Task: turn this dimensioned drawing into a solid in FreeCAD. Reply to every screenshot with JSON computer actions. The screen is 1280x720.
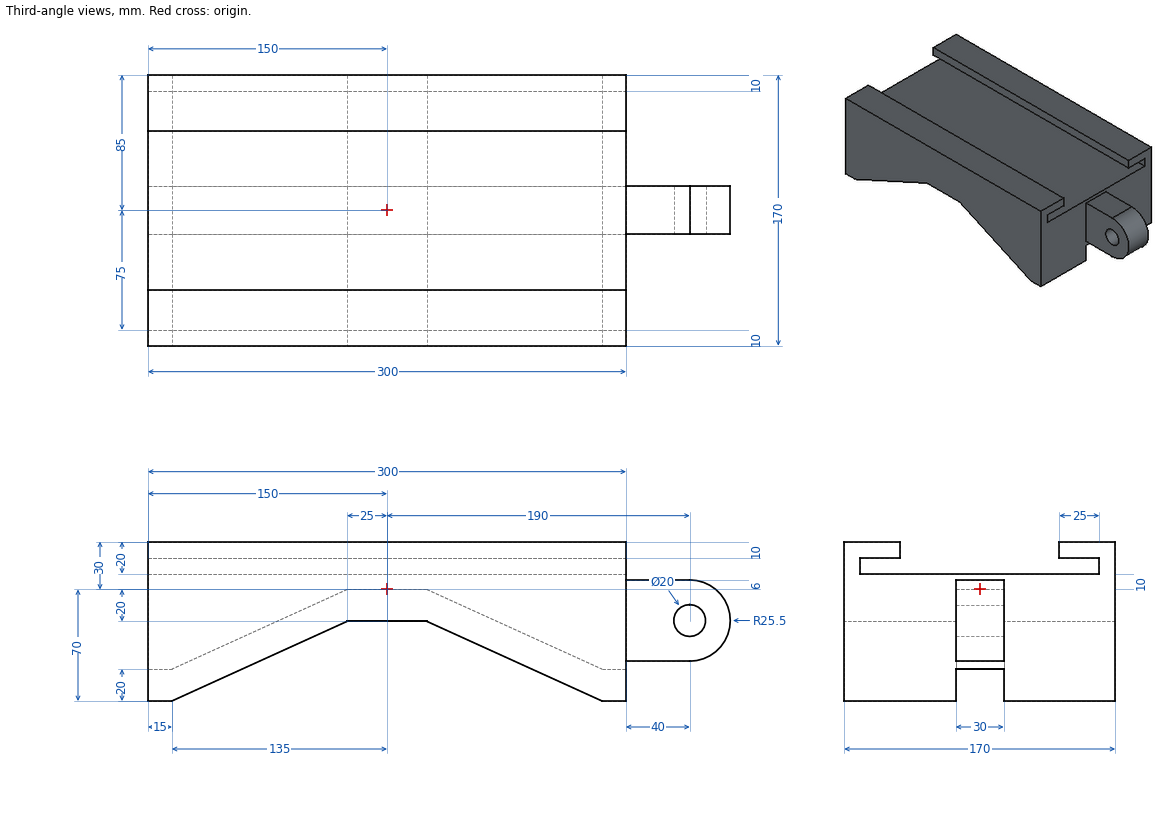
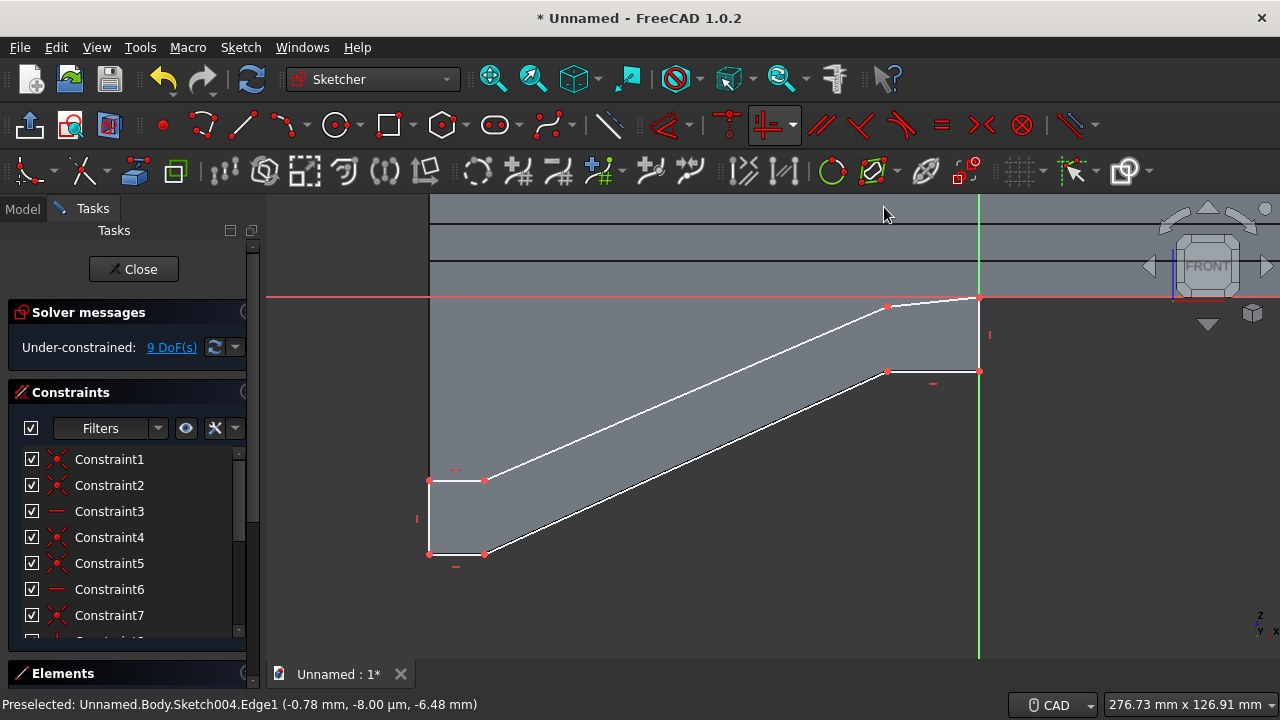
{"action": "left_click", "coordinate": [951, 300]}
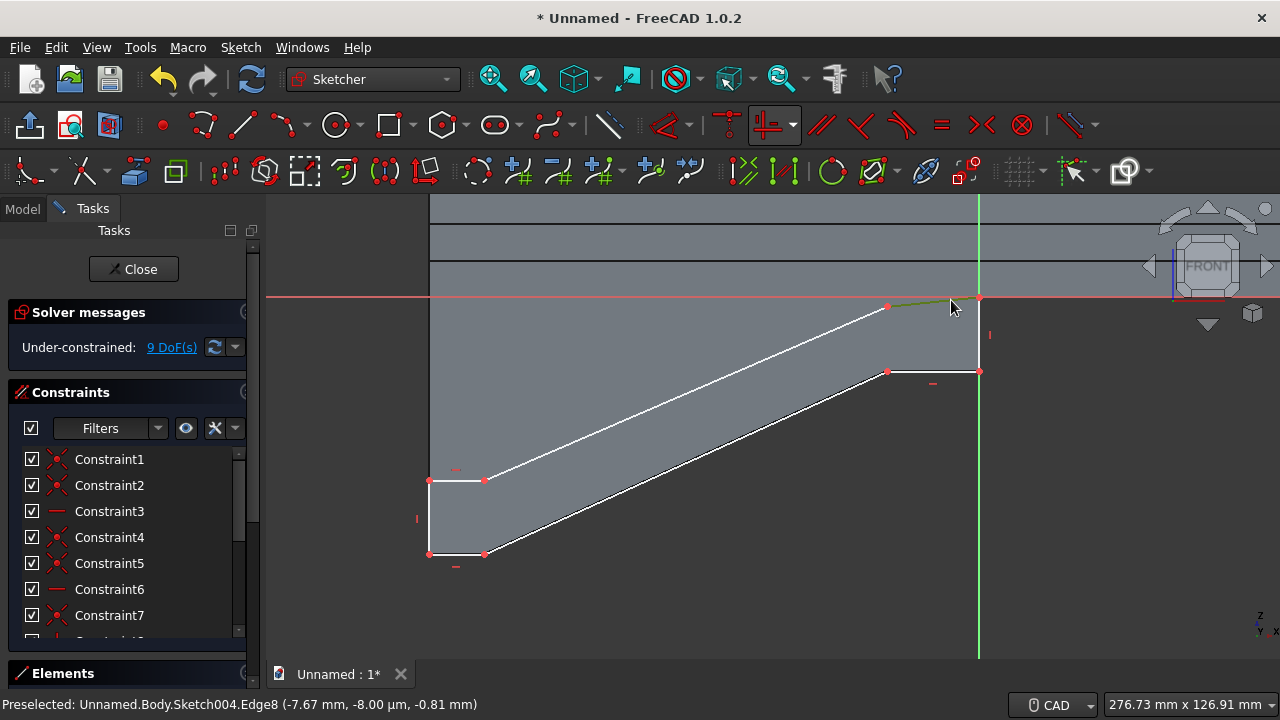
{"action": "key", "text": "h"}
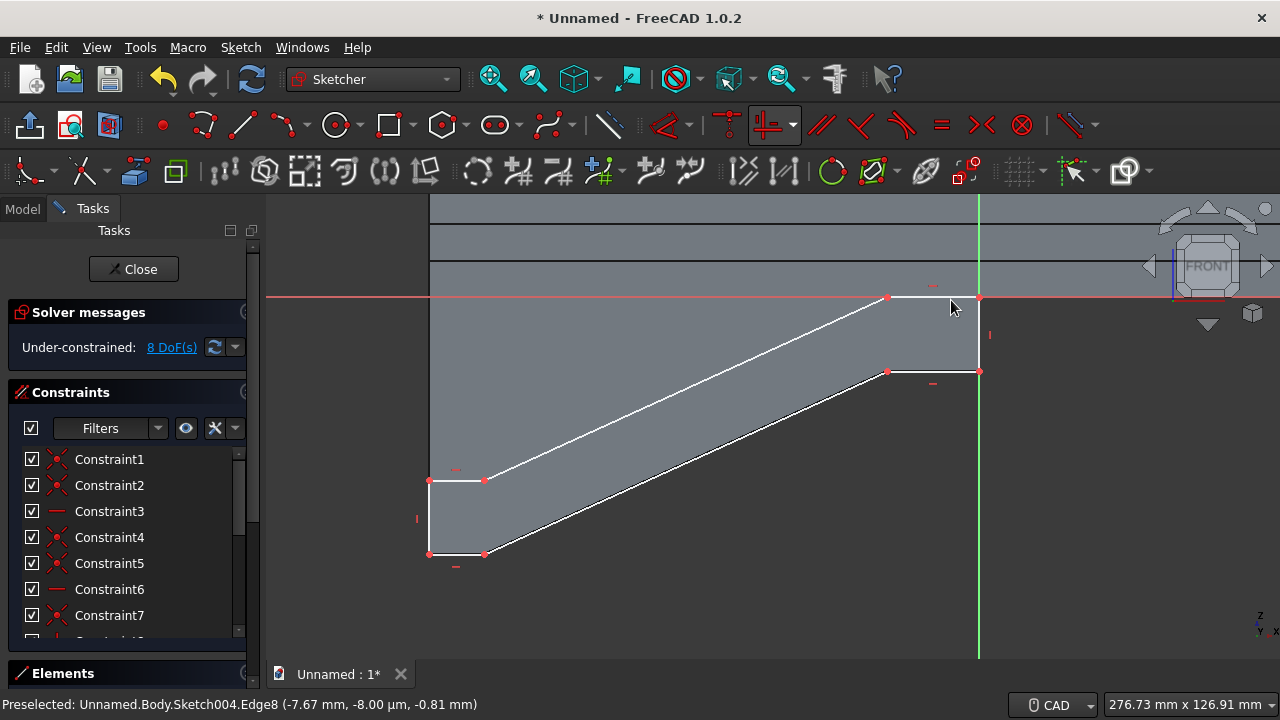
{"action": "key", "text": "d"}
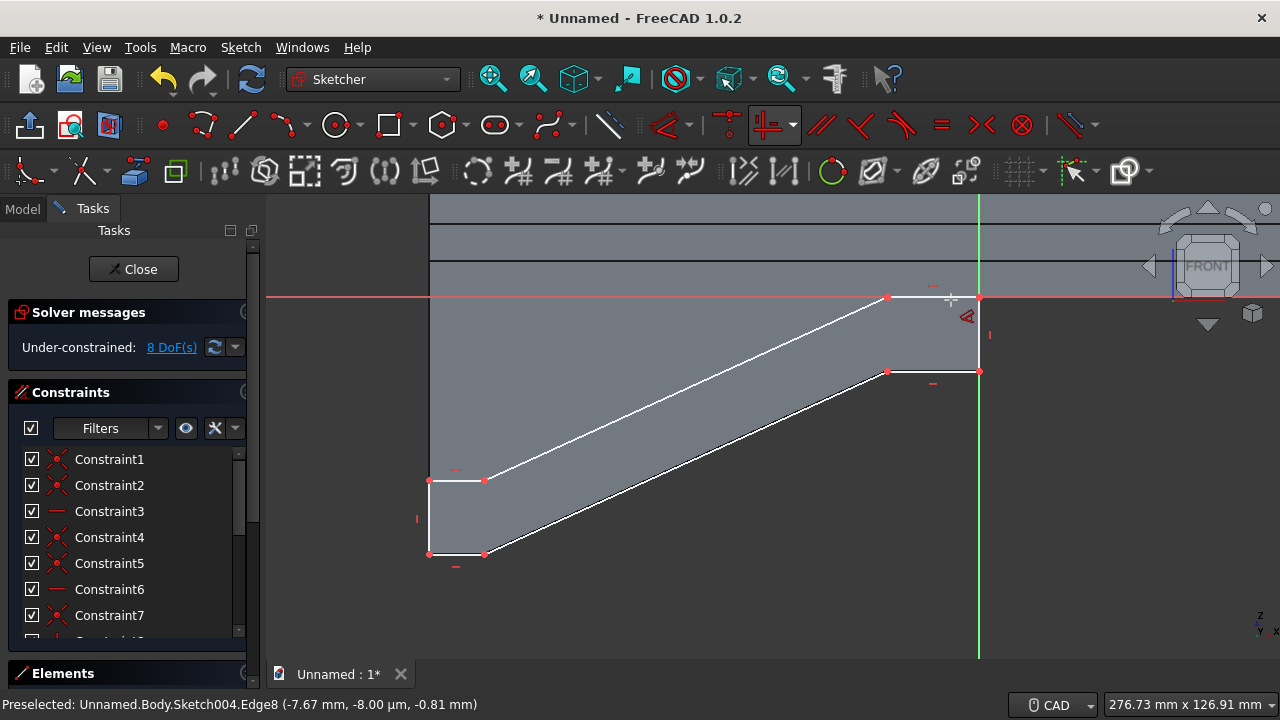
{"action": "left_click", "coordinate": [979, 320]}
{"action": "left_click", "coordinate": [1013, 335]}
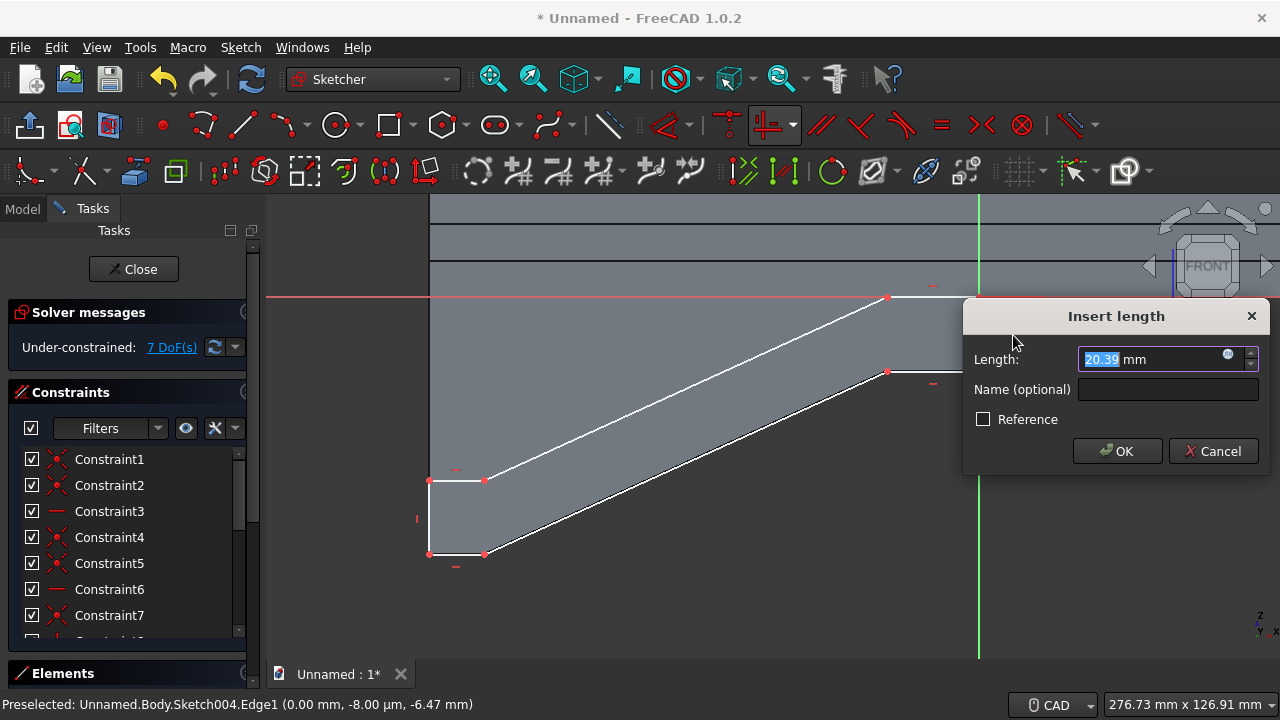
{"action": "type", "text": "20"}
{"action": "key", "text": "Return"}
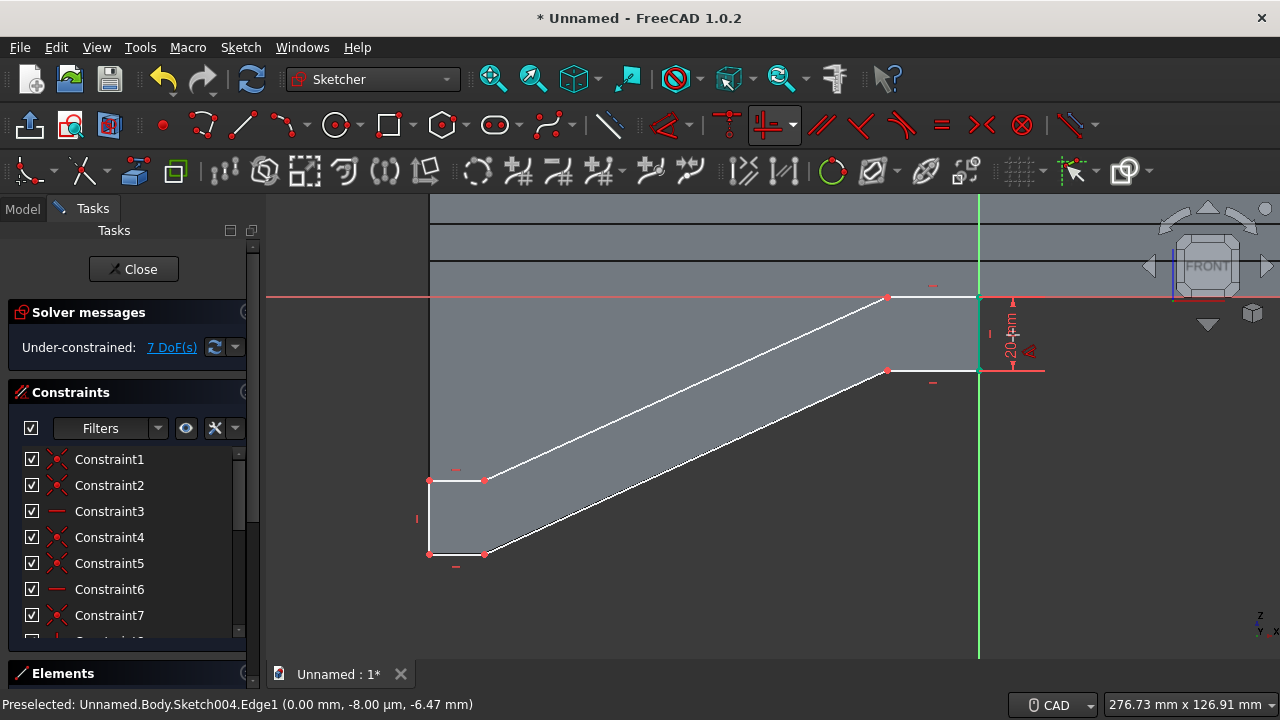
{"action": "left_click", "coordinate": [951, 371]}
{"action": "left_click", "coordinate": [933, 337]}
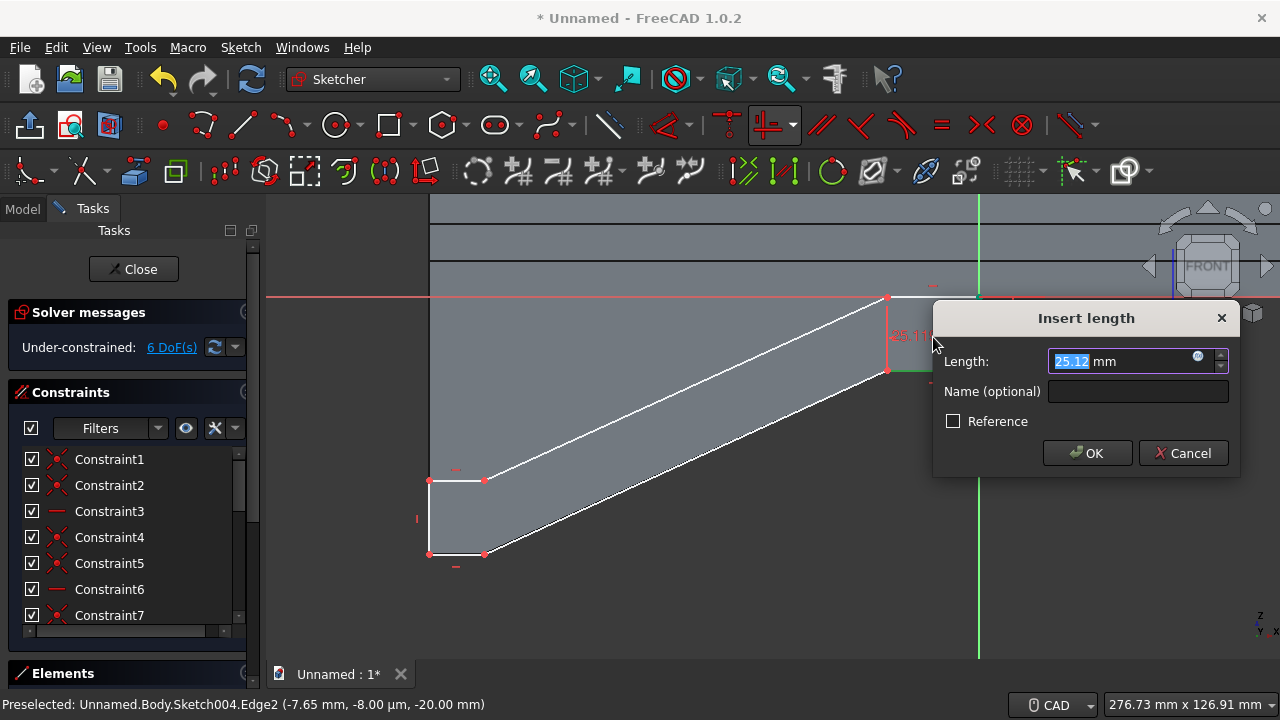
{"action": "type", "text": "25"}
{"action": "key", "text": "Return"}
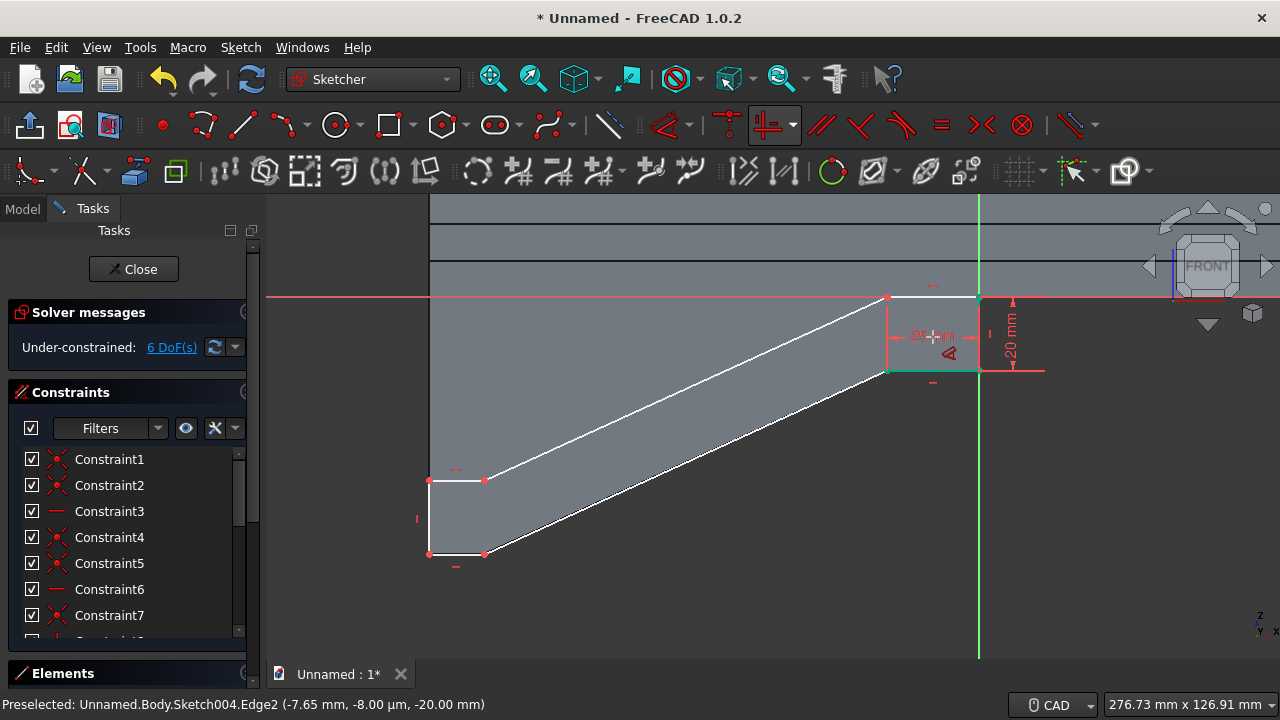
{"action": "left_click", "coordinate": [468, 555]}
{"action": "left_click", "coordinate": [457, 589]}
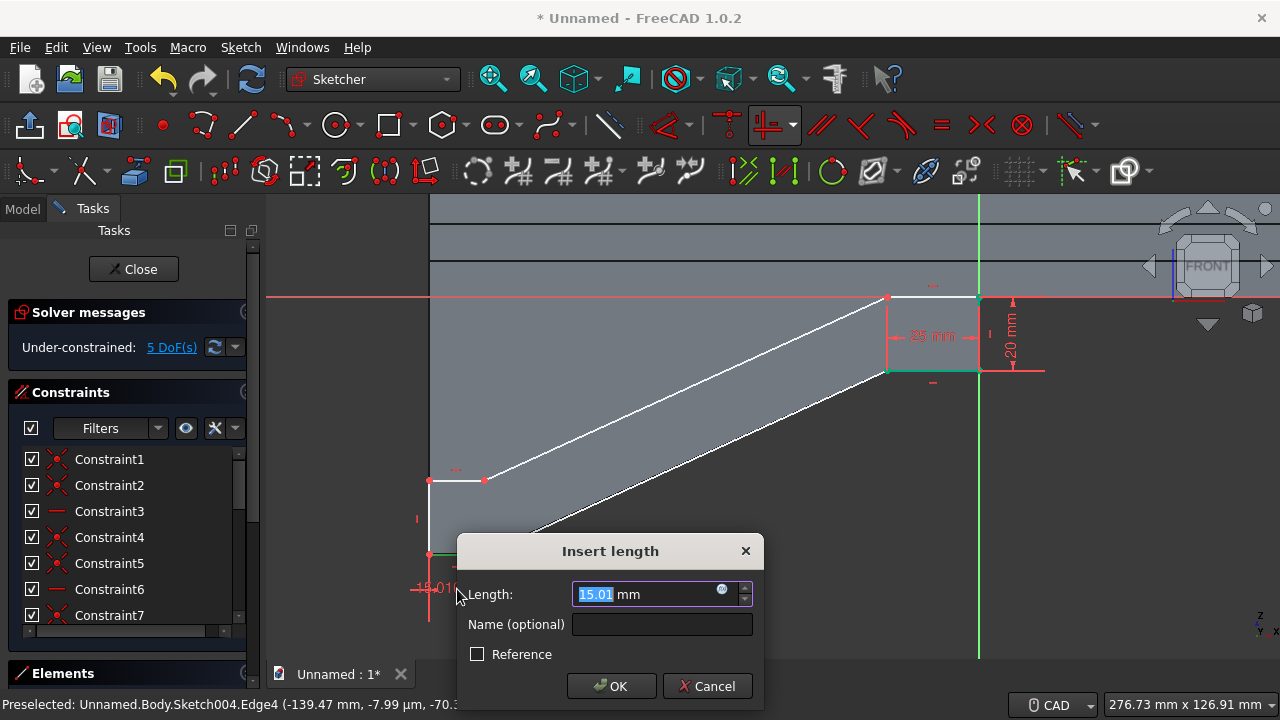
{"action": "type", "text": "15"}
{"action": "key", "text": "Return"}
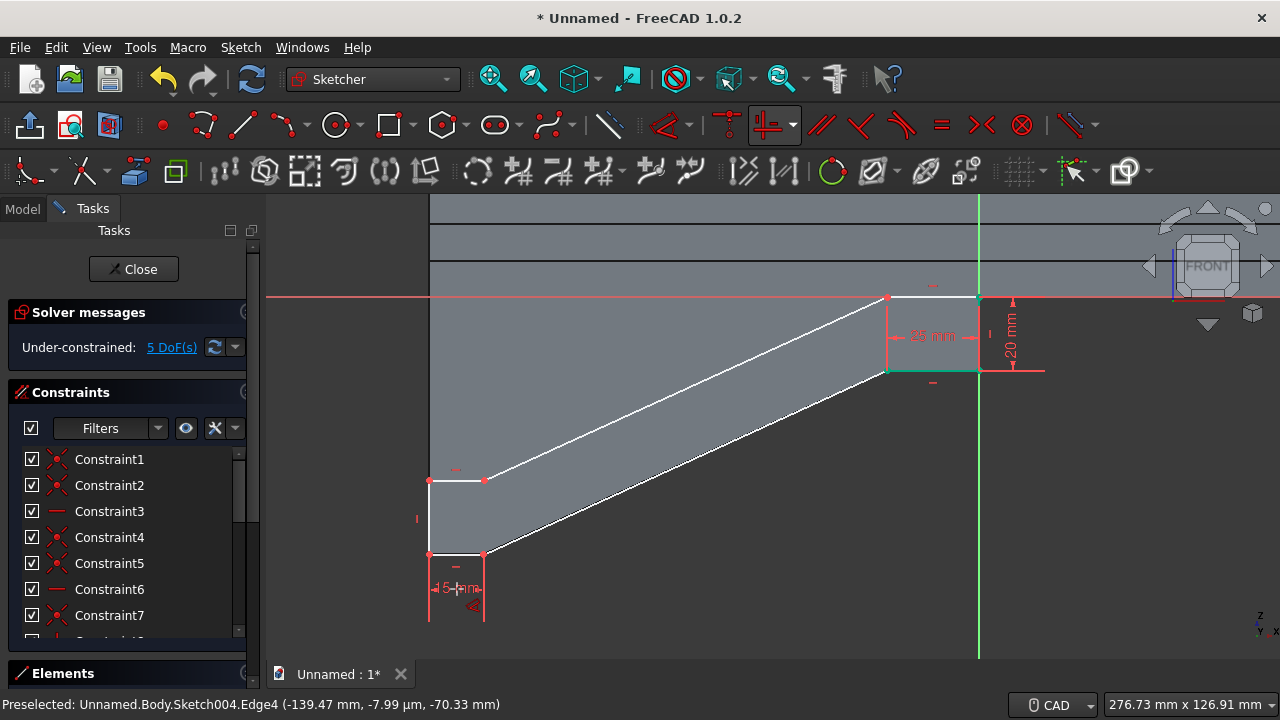
{"action": "left_click", "coordinate": [429, 533]}
{"action": "left_click", "coordinate": [395, 518]}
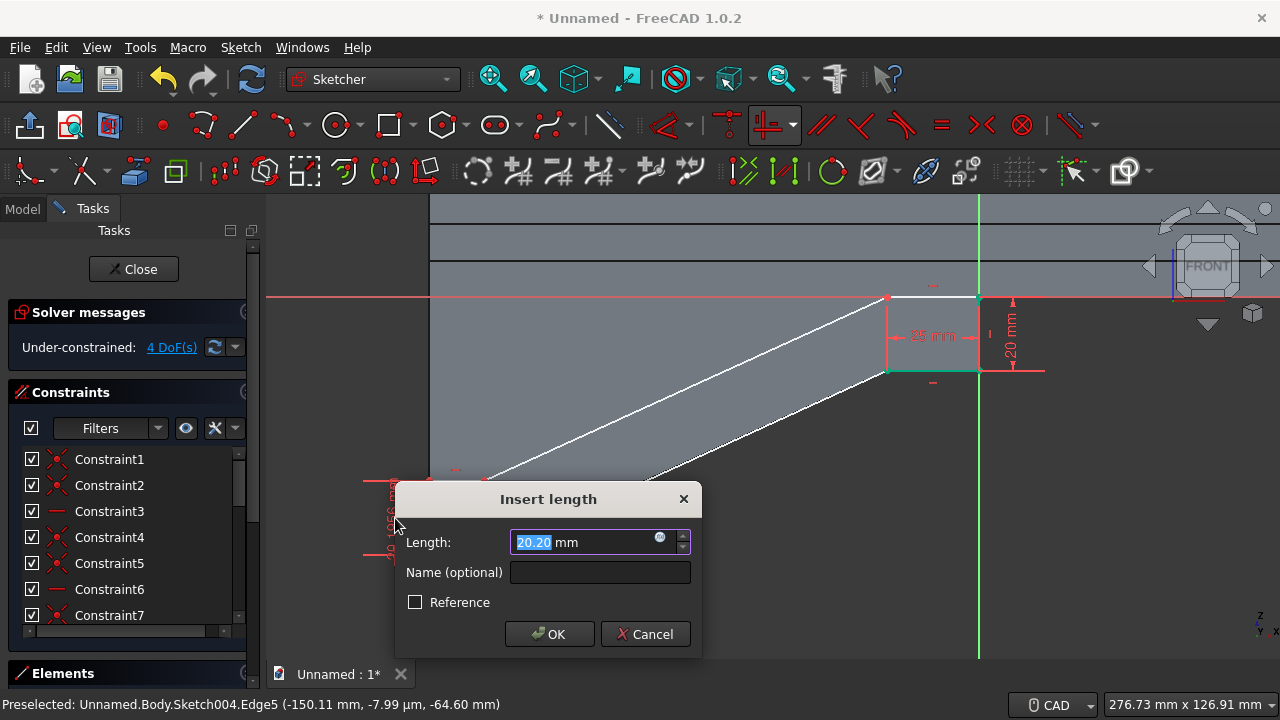
{"action": "type", "text": "20"}
{"action": "key", "text": "Return"}